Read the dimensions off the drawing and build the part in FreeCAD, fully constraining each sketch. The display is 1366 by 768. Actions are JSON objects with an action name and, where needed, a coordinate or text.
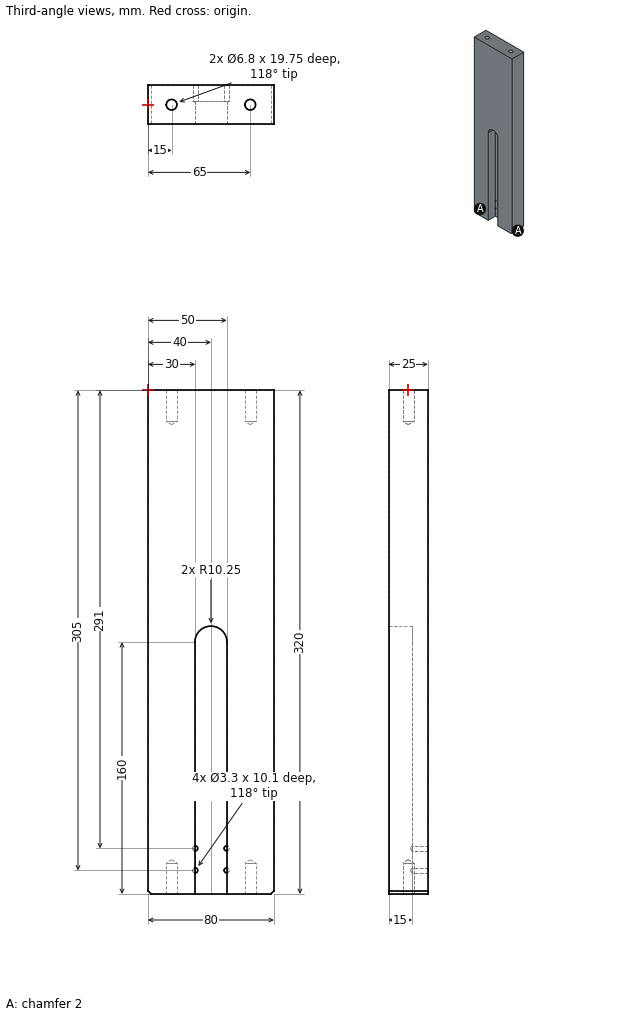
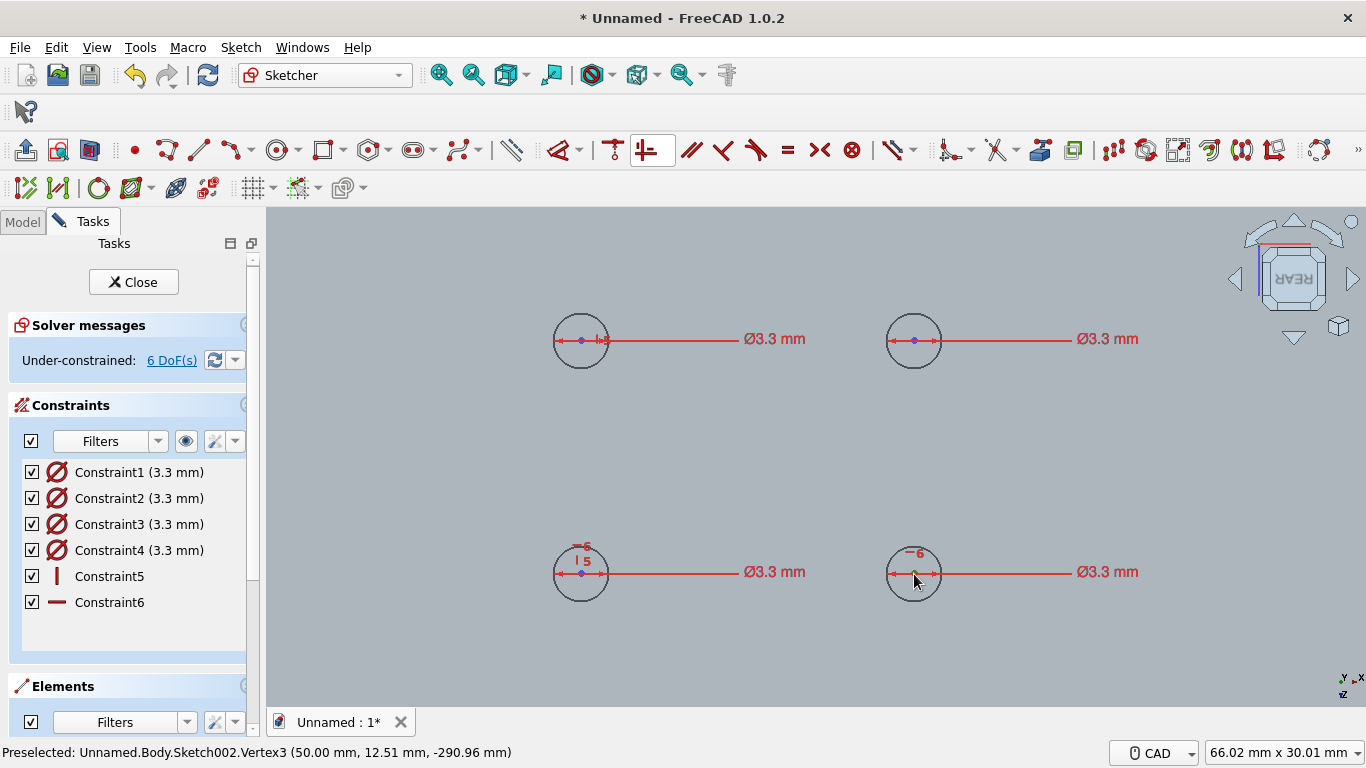
{"action": "left_click", "coordinate": [914, 341]}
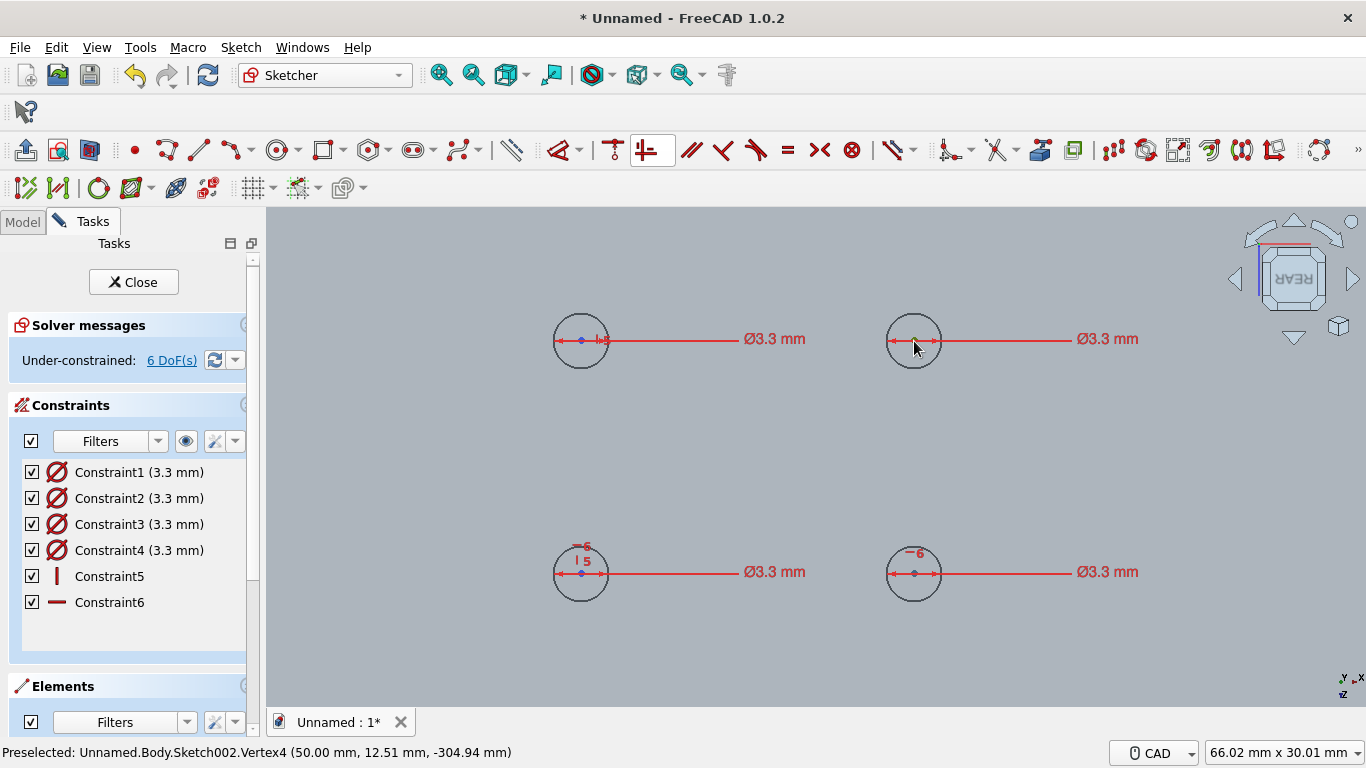
{"action": "left_click", "coordinate": [670, 150]}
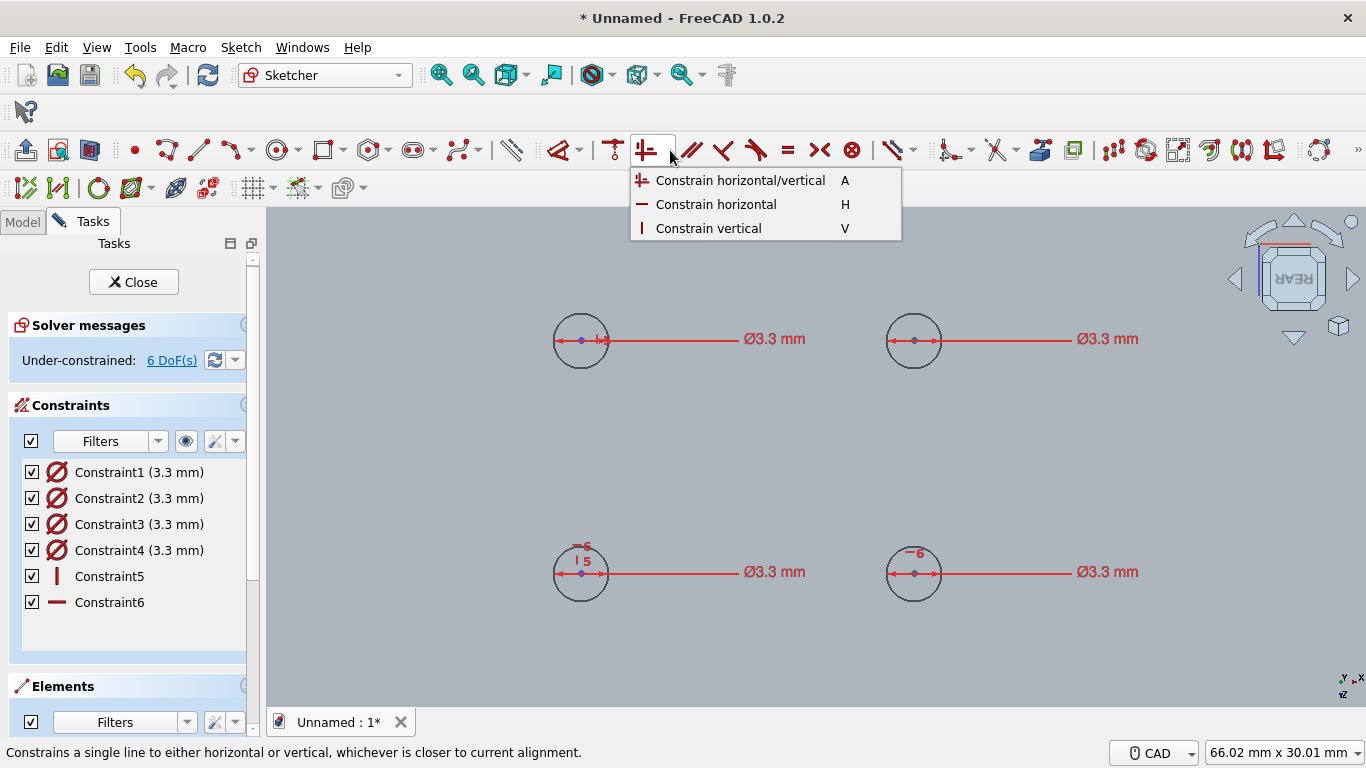
{"action": "left_click", "coordinate": [766, 228]}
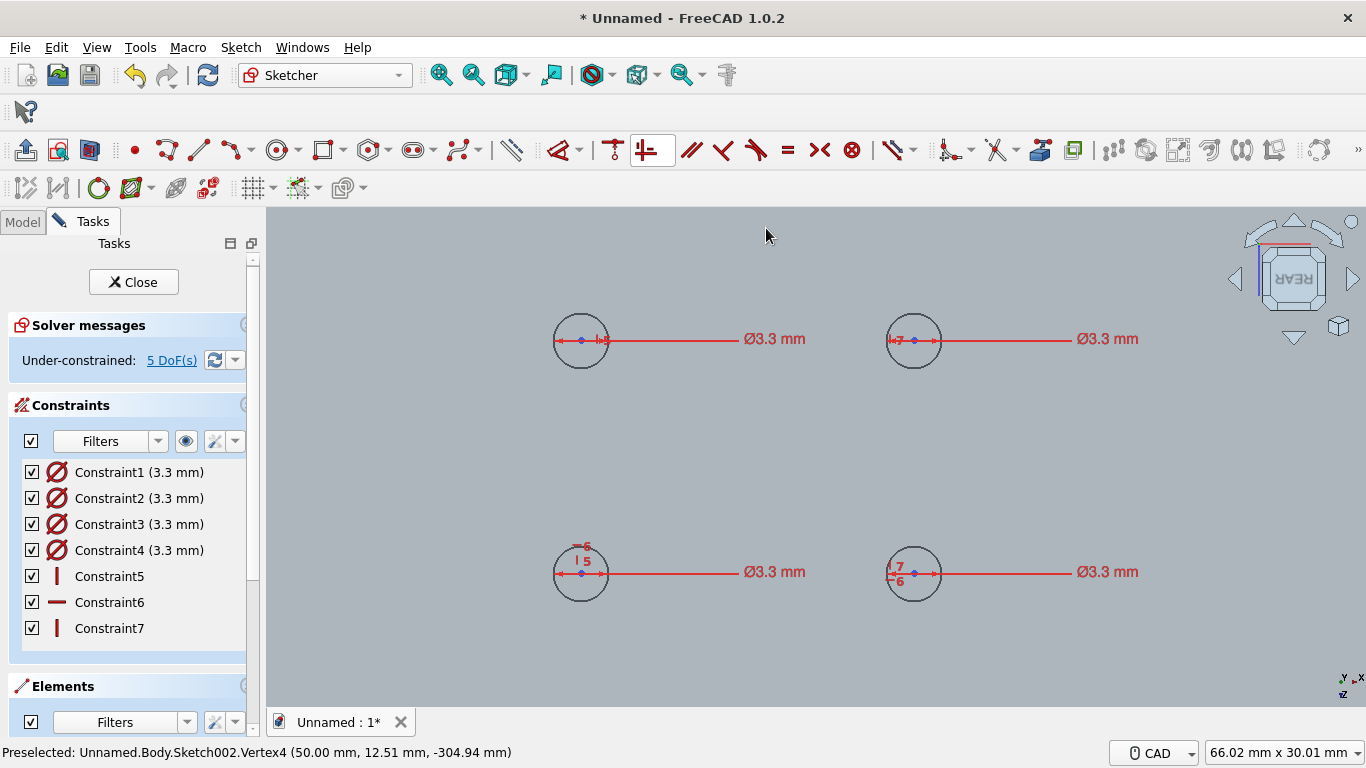
{"action": "left_click", "coordinate": [581, 341]}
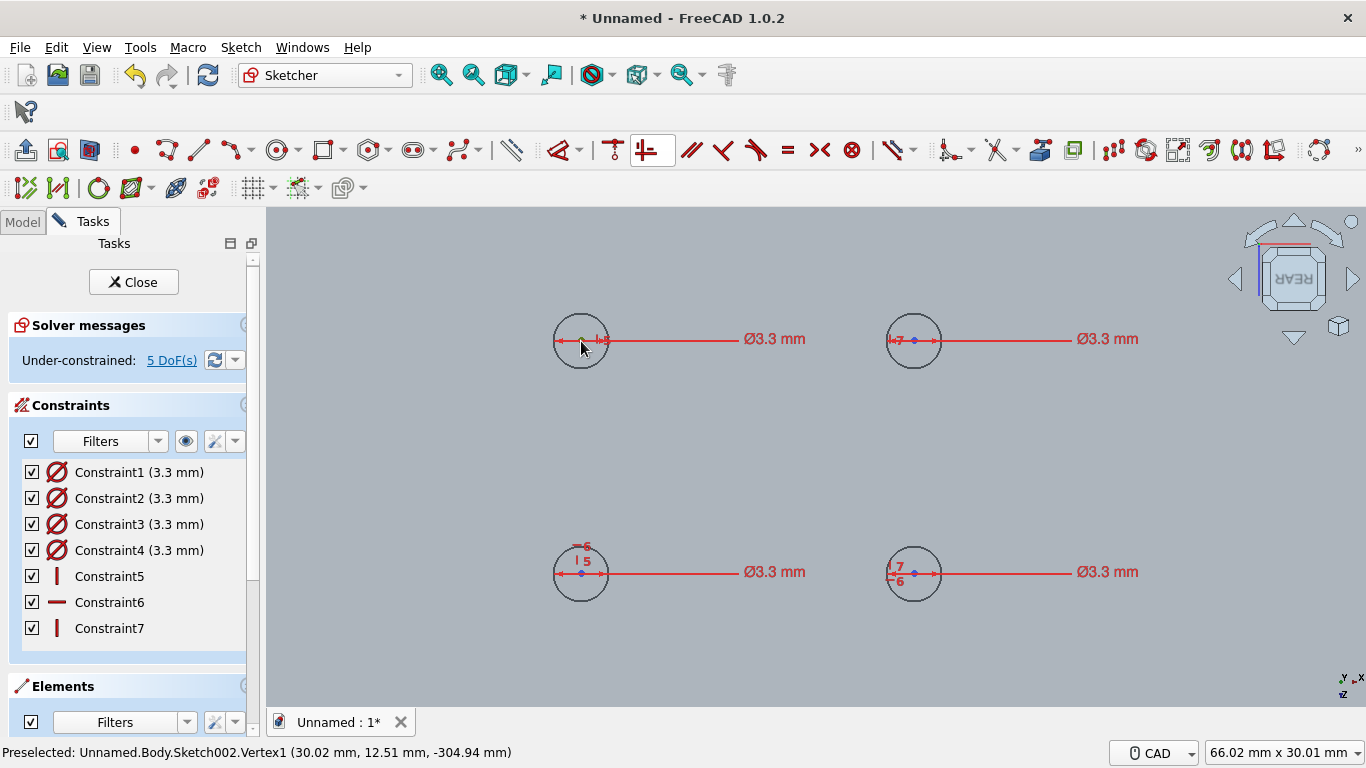
{"action": "left_click", "coordinate": [914, 341]}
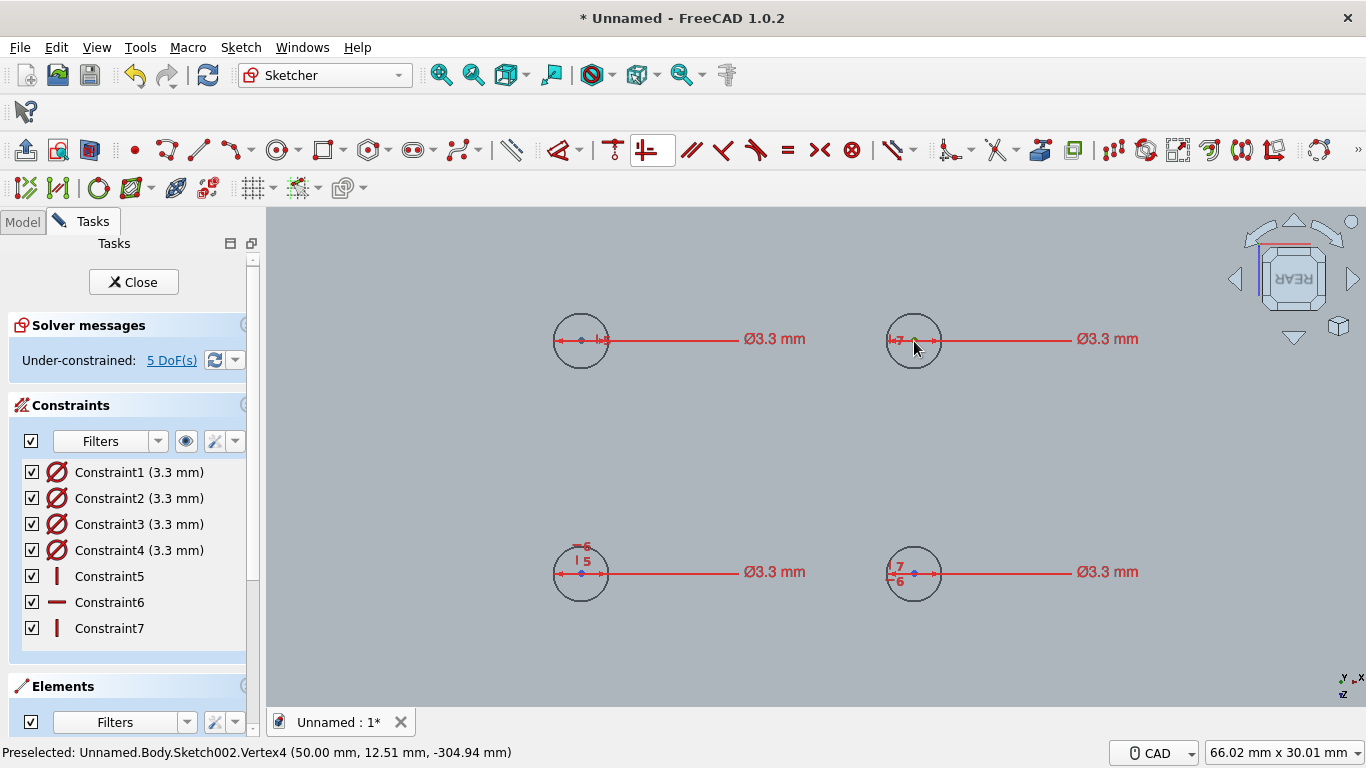
{"action": "key", "text": "h"}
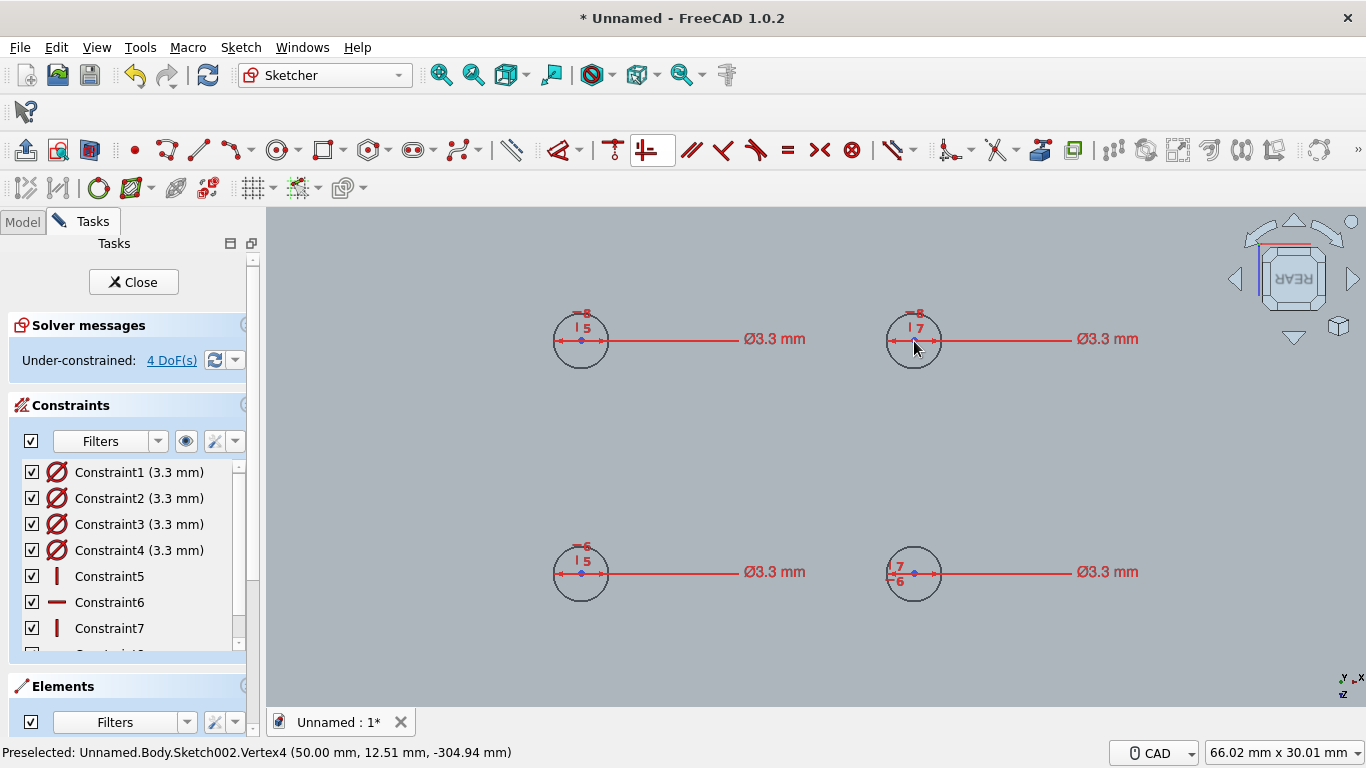
{"action": "left_click", "coordinate": [558, 150]}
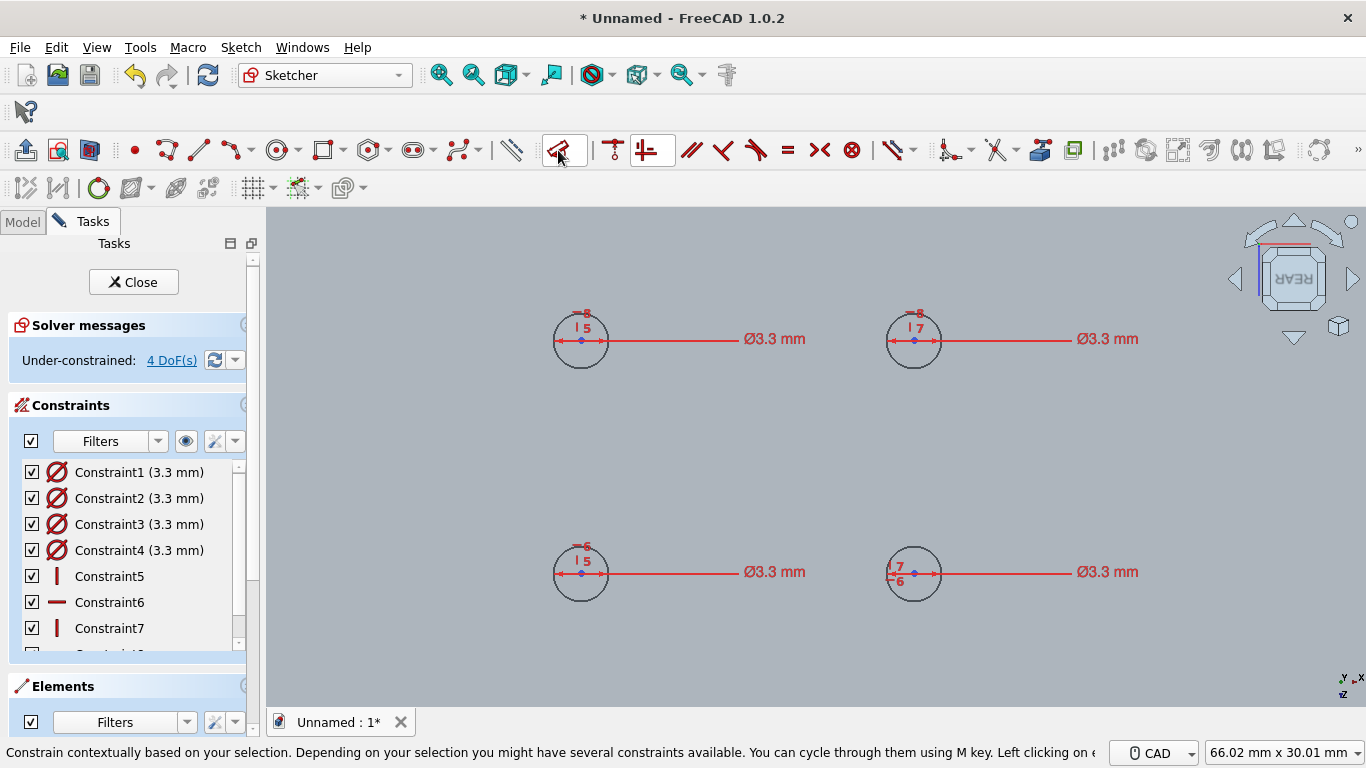
{"action": "left_click", "coordinate": [581, 341]}
{"action": "left_click", "coordinate": [438, 307]}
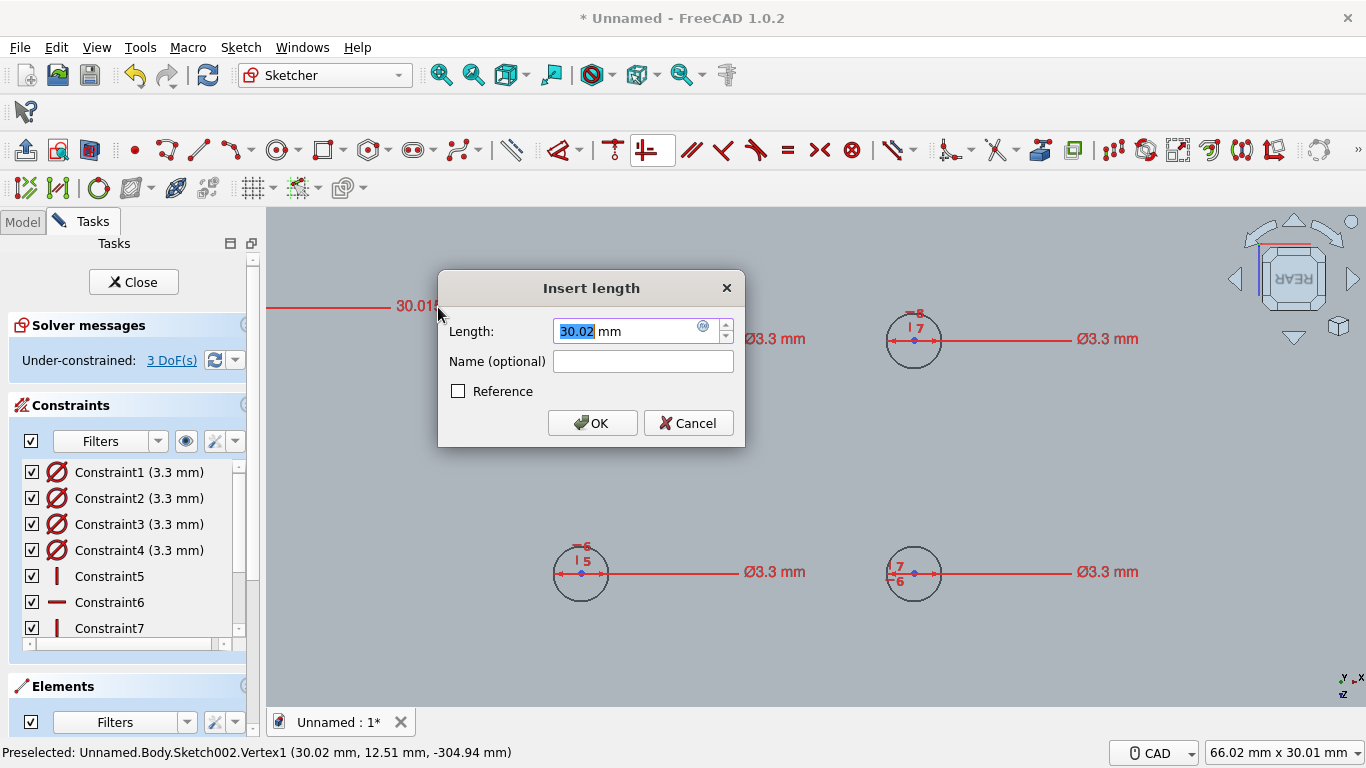
{"action": "type", "text": "30"}
{"action": "key", "text": "Return"}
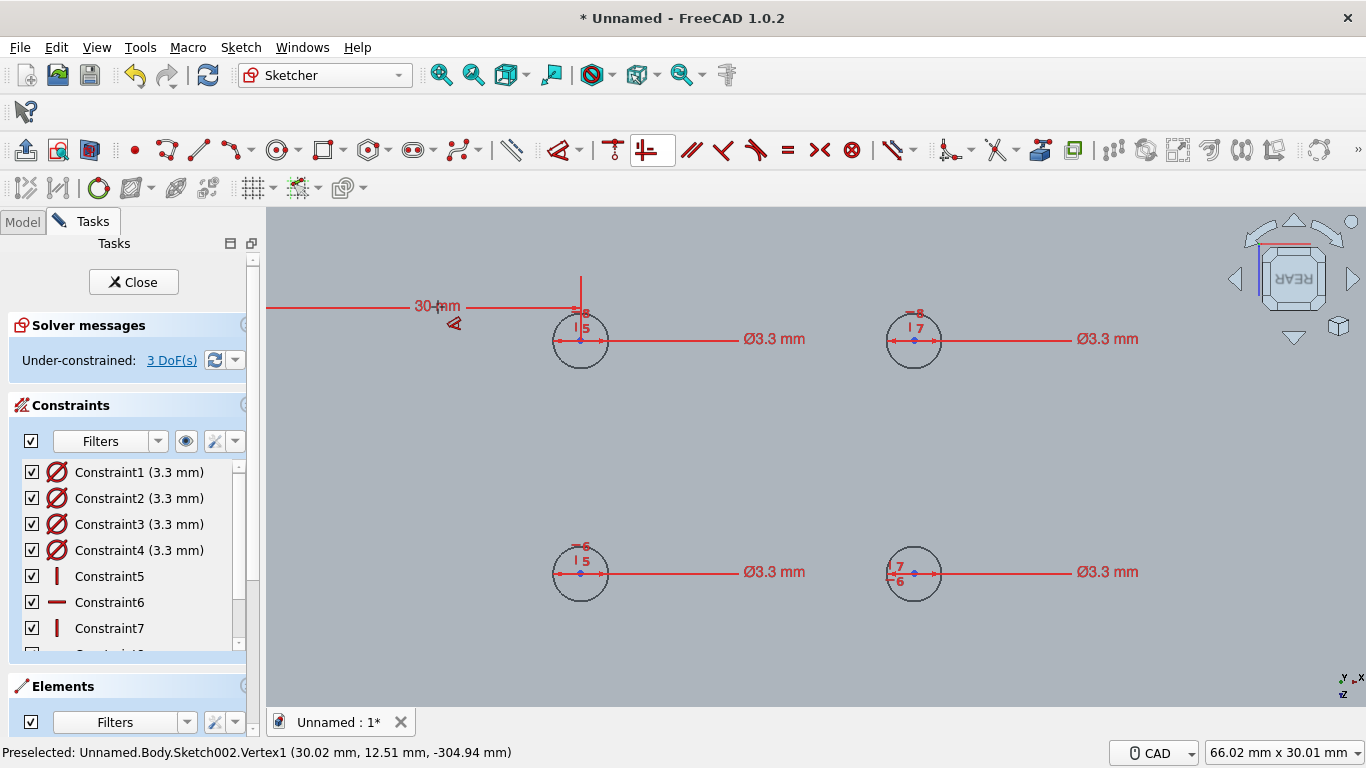
{"action": "left_click", "coordinate": [914, 574]}
{"action": "left_click", "coordinate": [604, 540]}